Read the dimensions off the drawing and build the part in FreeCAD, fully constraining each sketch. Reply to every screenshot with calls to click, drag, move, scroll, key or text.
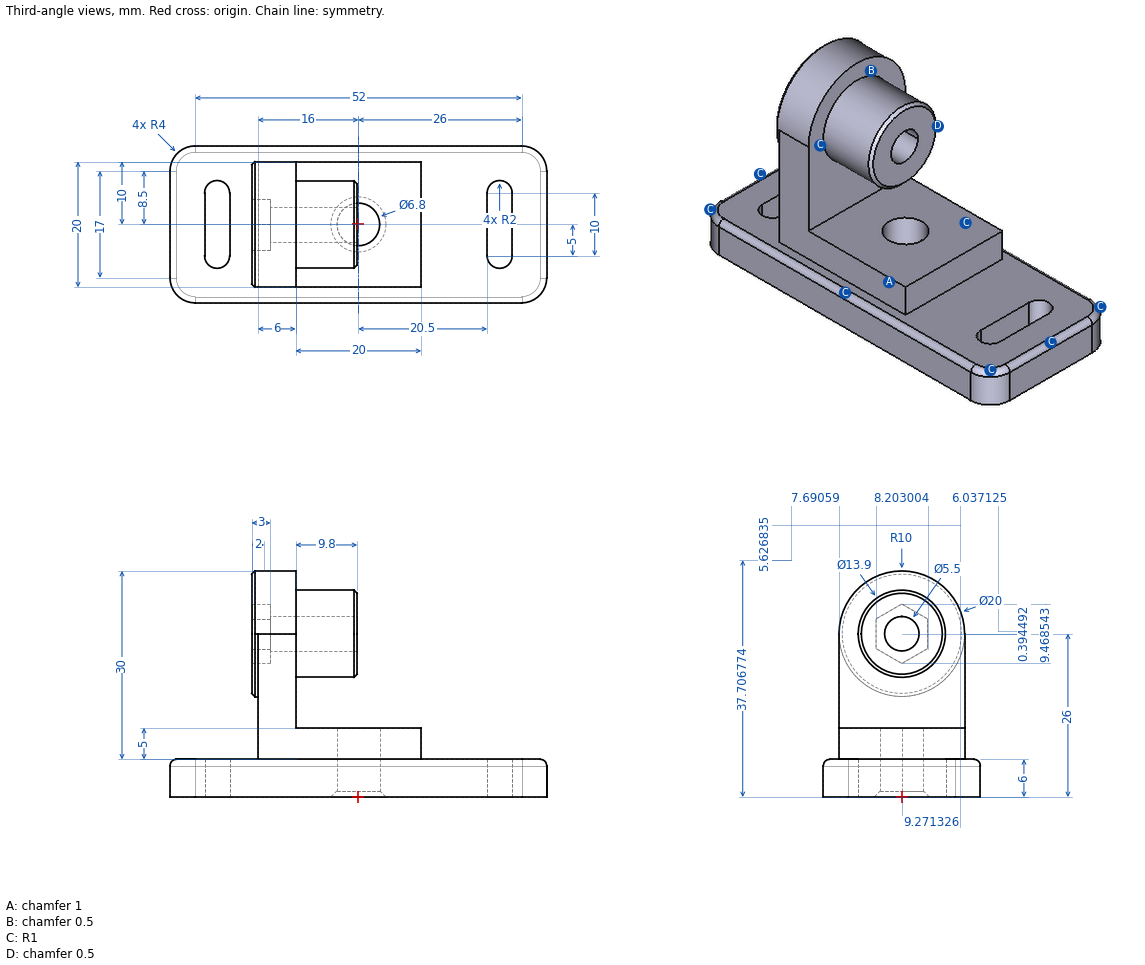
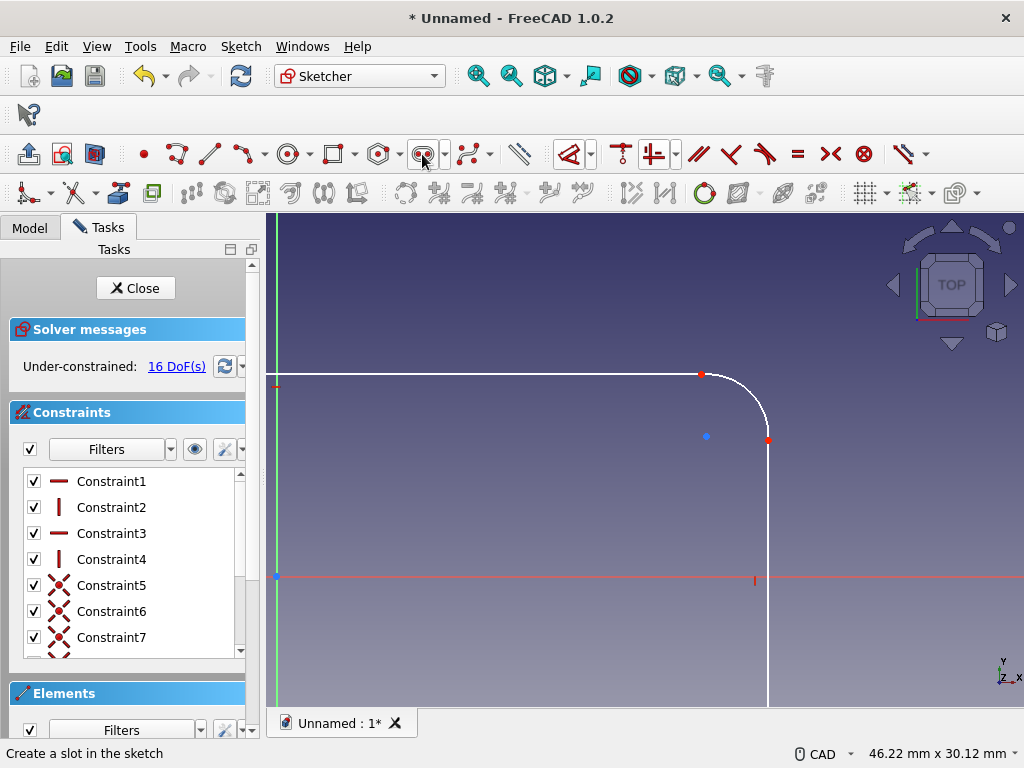
click(646, 659)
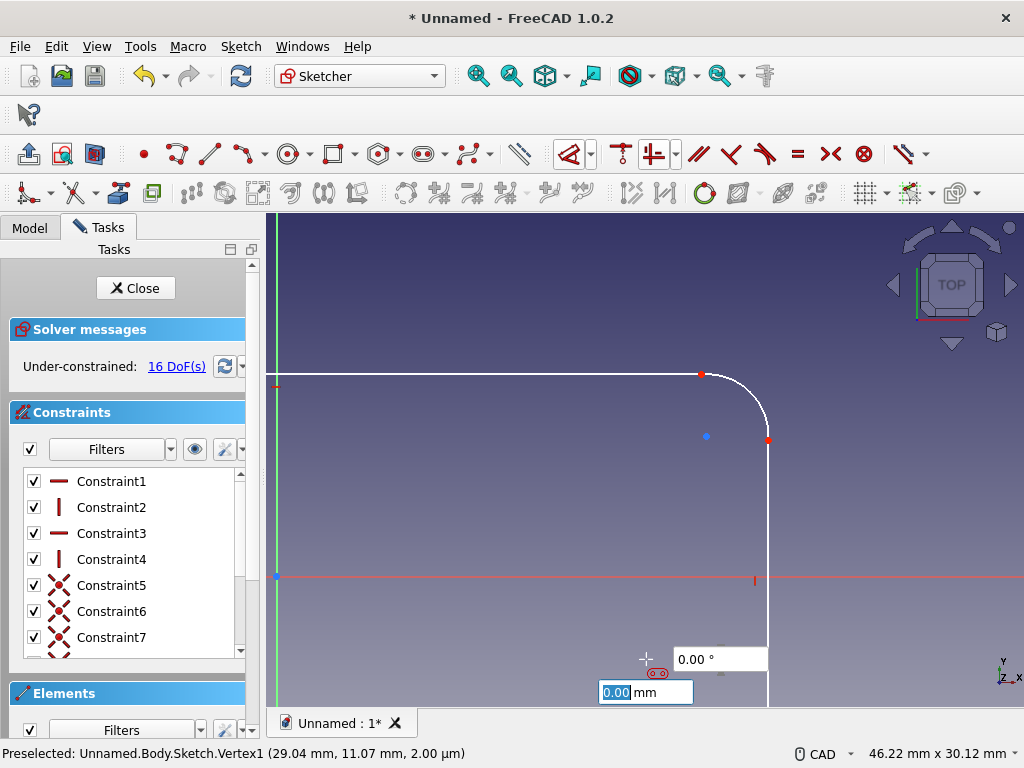
click(646, 495)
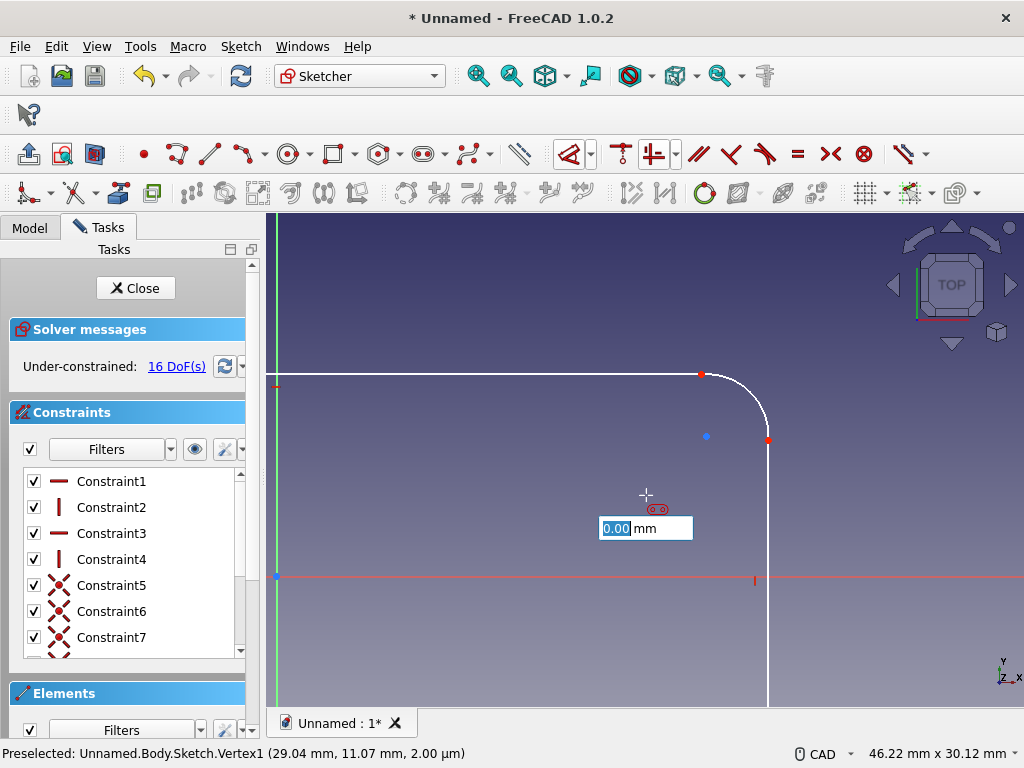
click(679, 552)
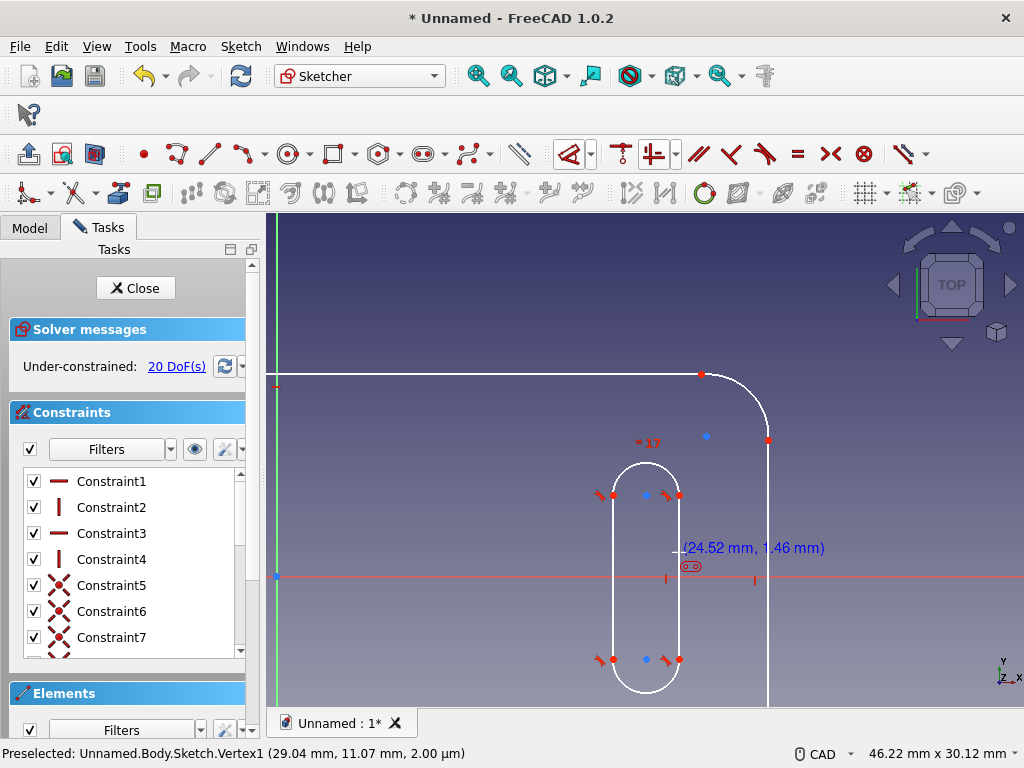
scroll(751, 392, down, 5)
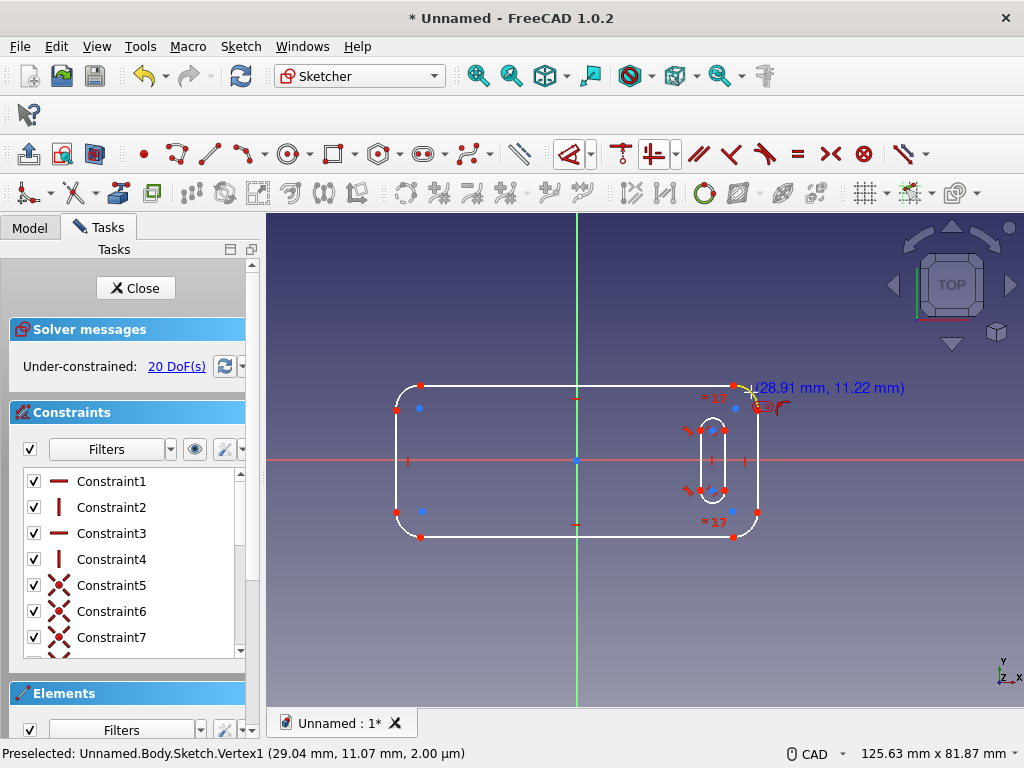
scroll(441, 490, up, 4)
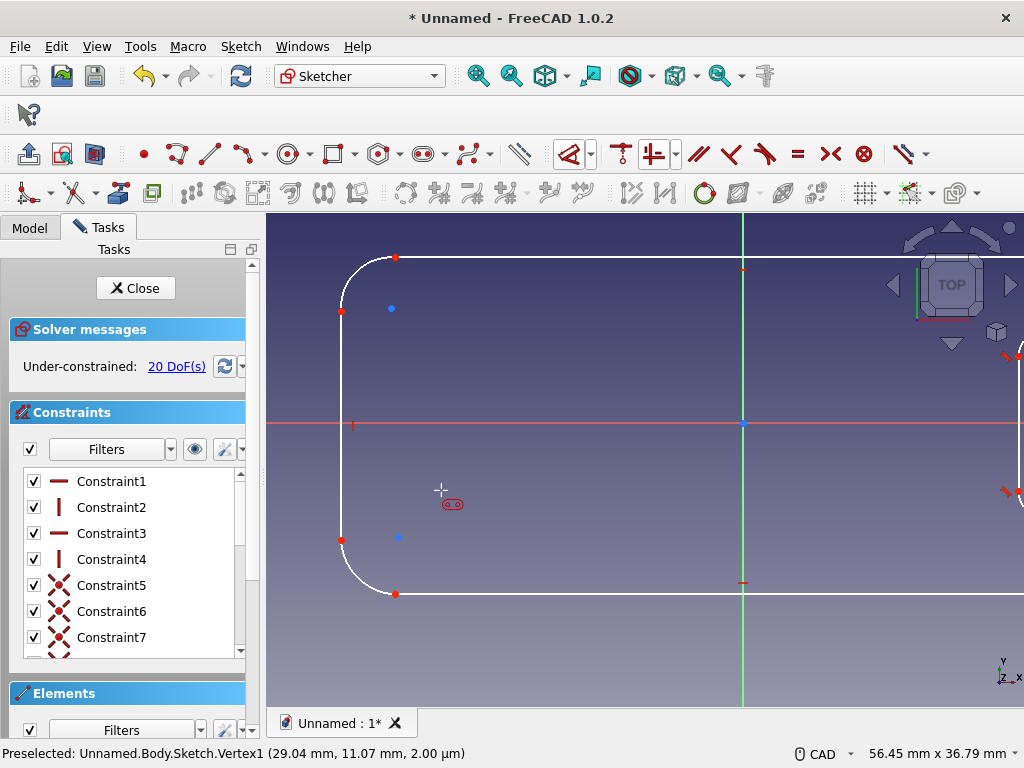
click(441, 490)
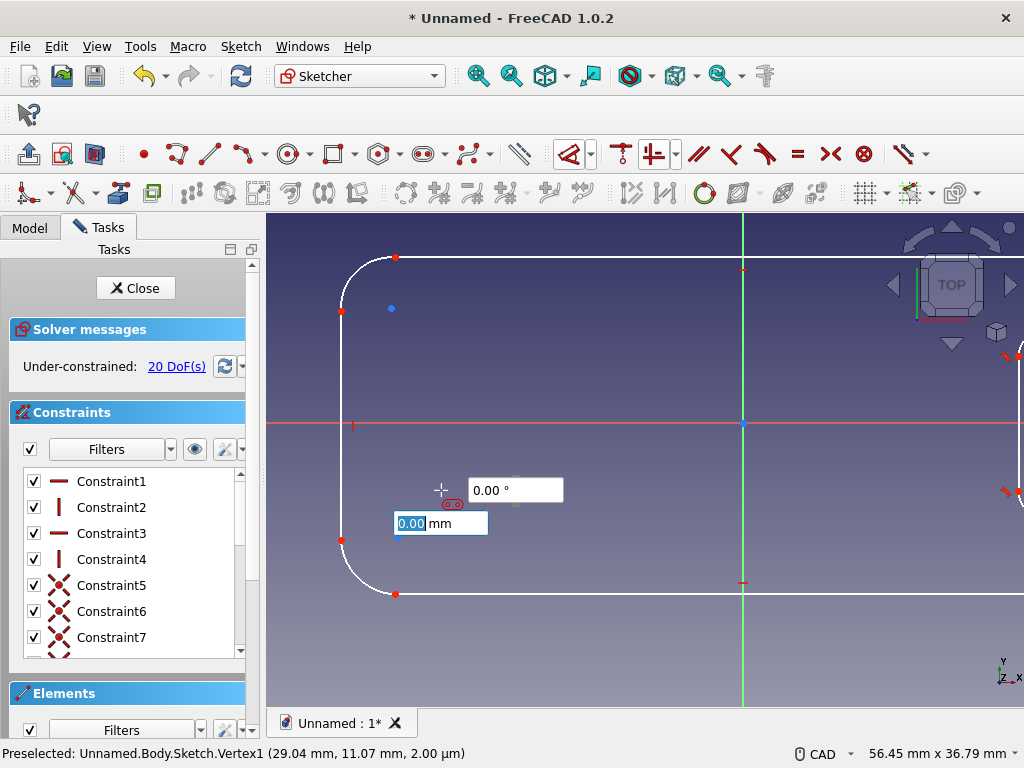
click(441, 356)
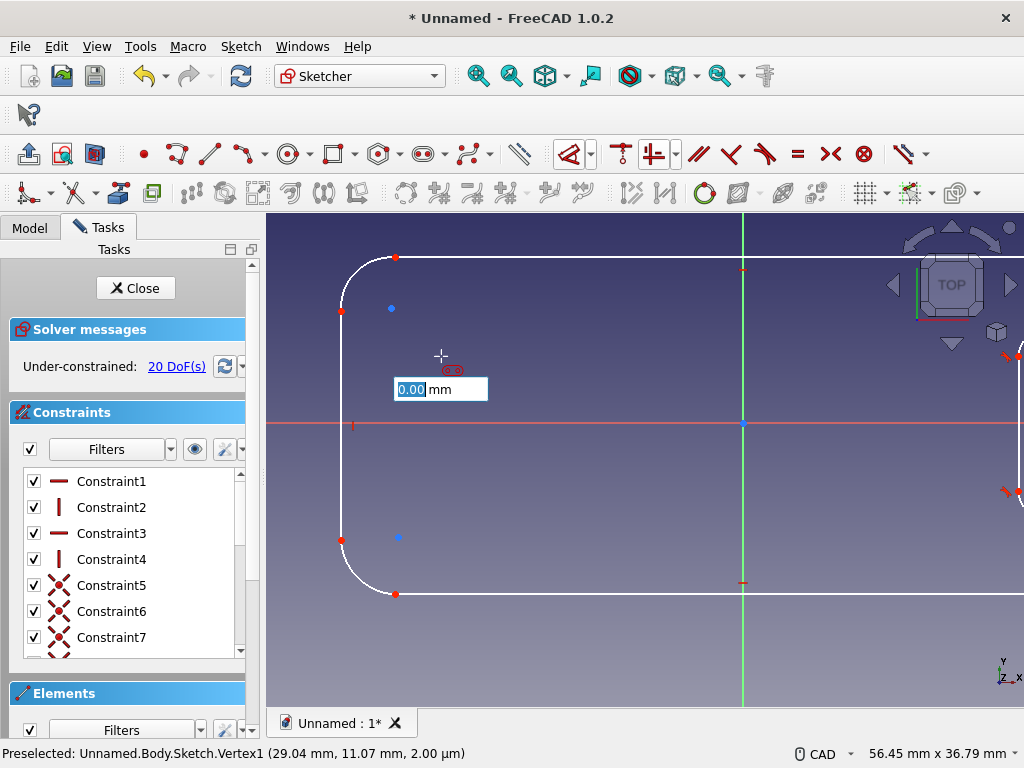
click(468, 403)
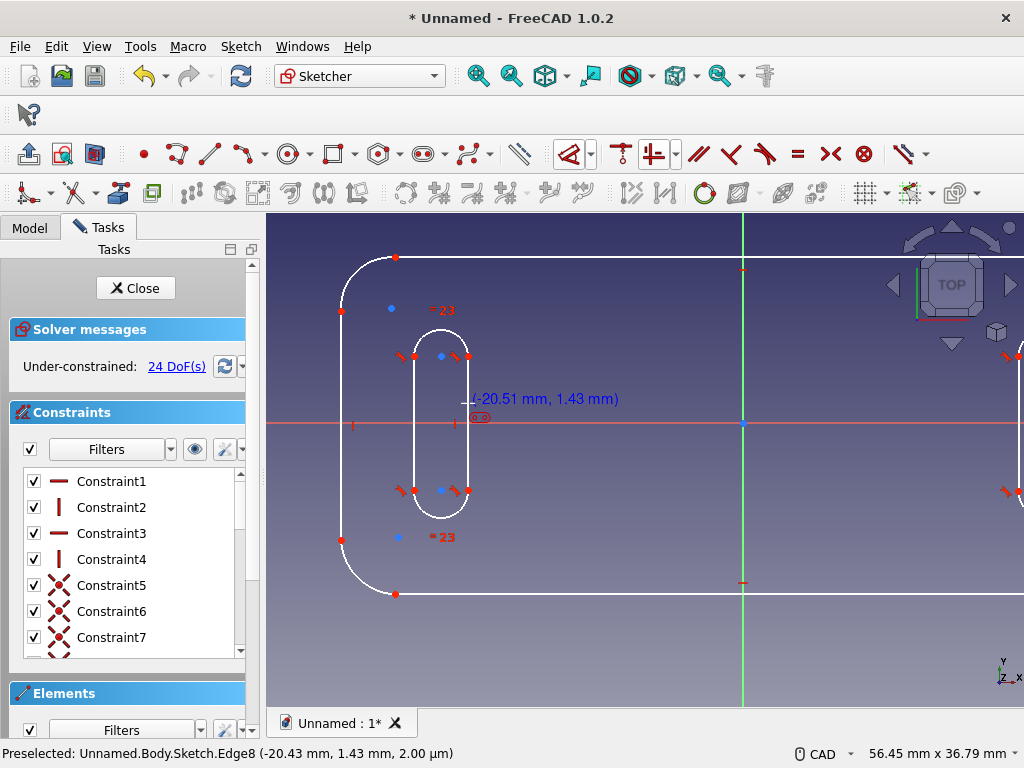
key(g)
key(c)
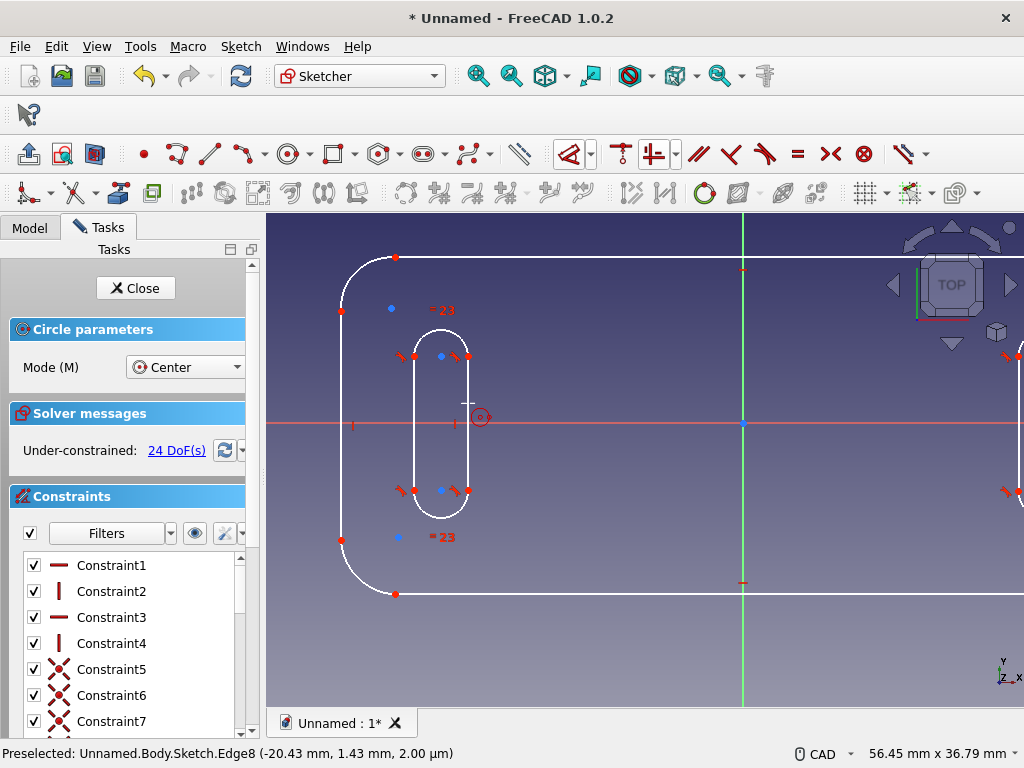
click(743, 423)
move(776, 391)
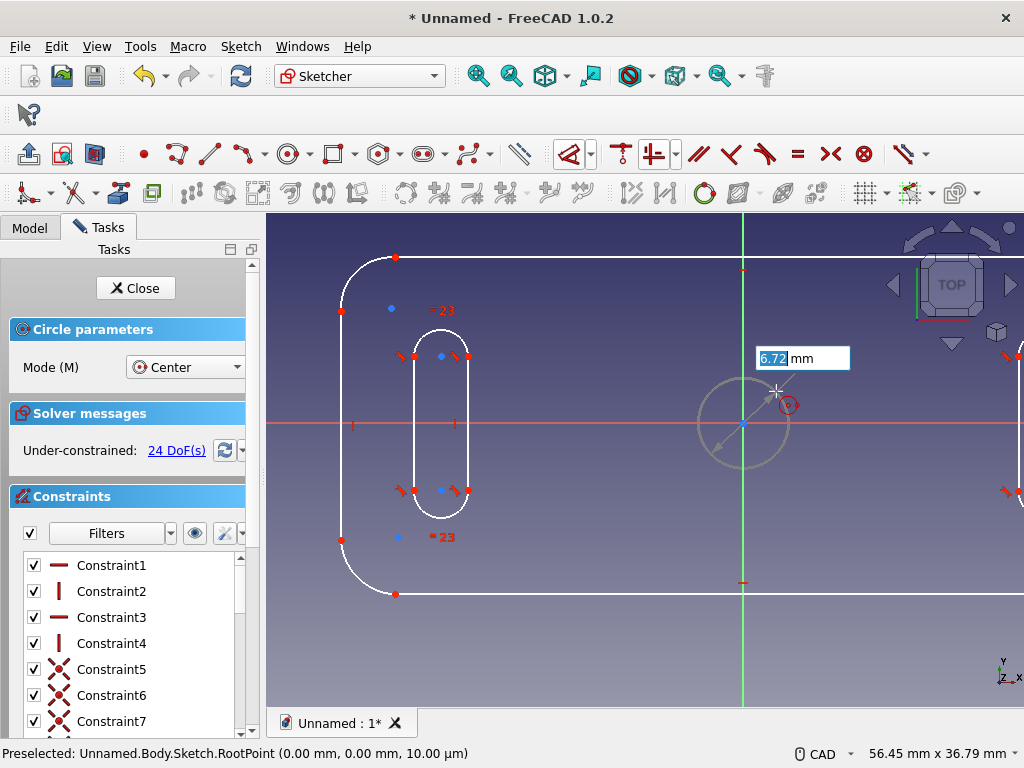
text(6.8)
key(Return)
key(Escape)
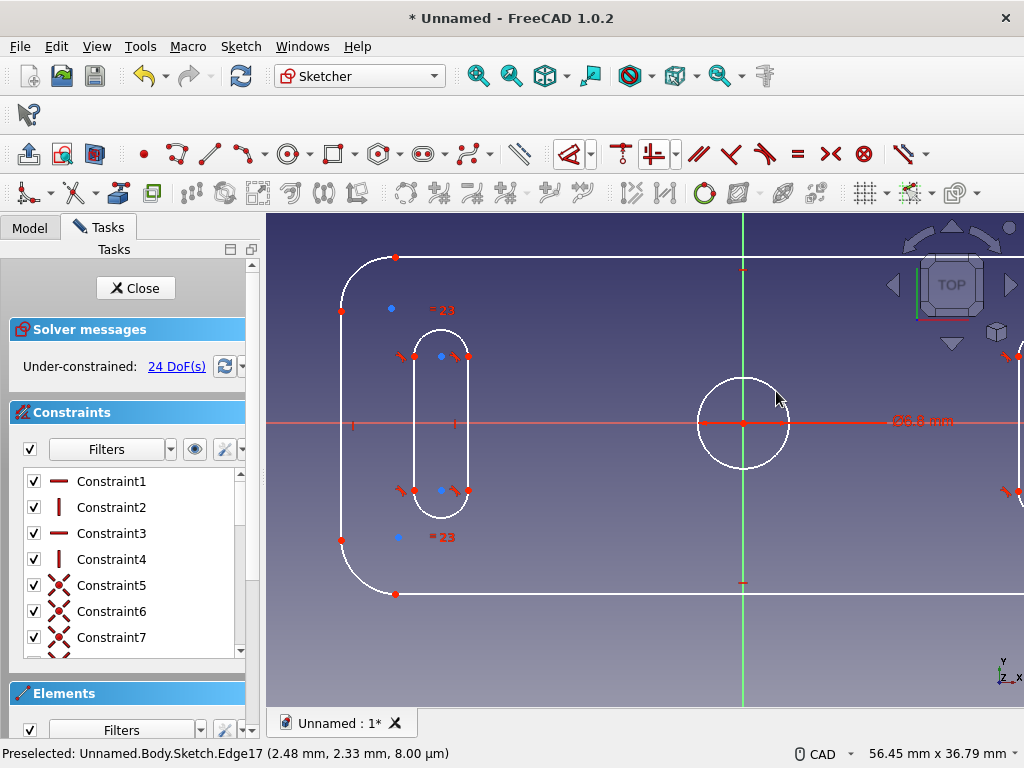
click(604, 257)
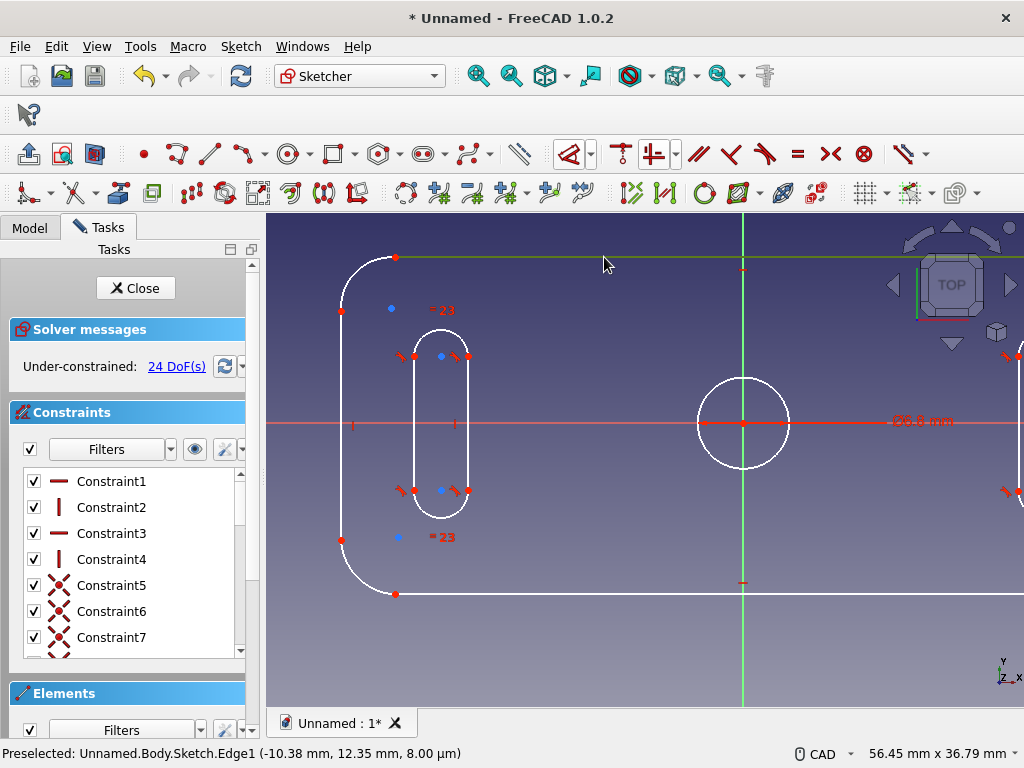
click(370, 262)